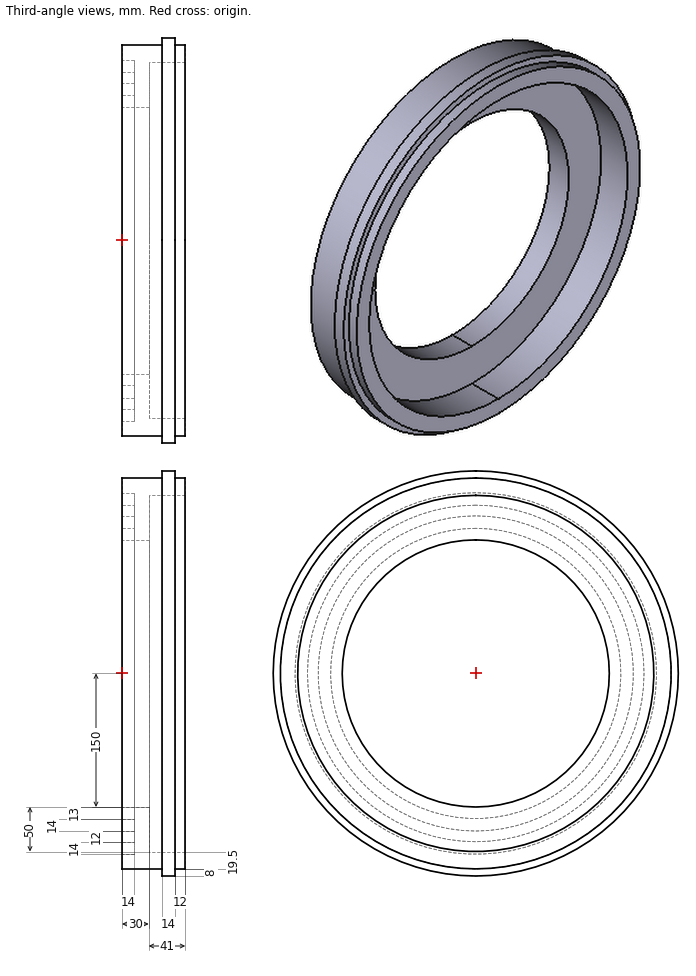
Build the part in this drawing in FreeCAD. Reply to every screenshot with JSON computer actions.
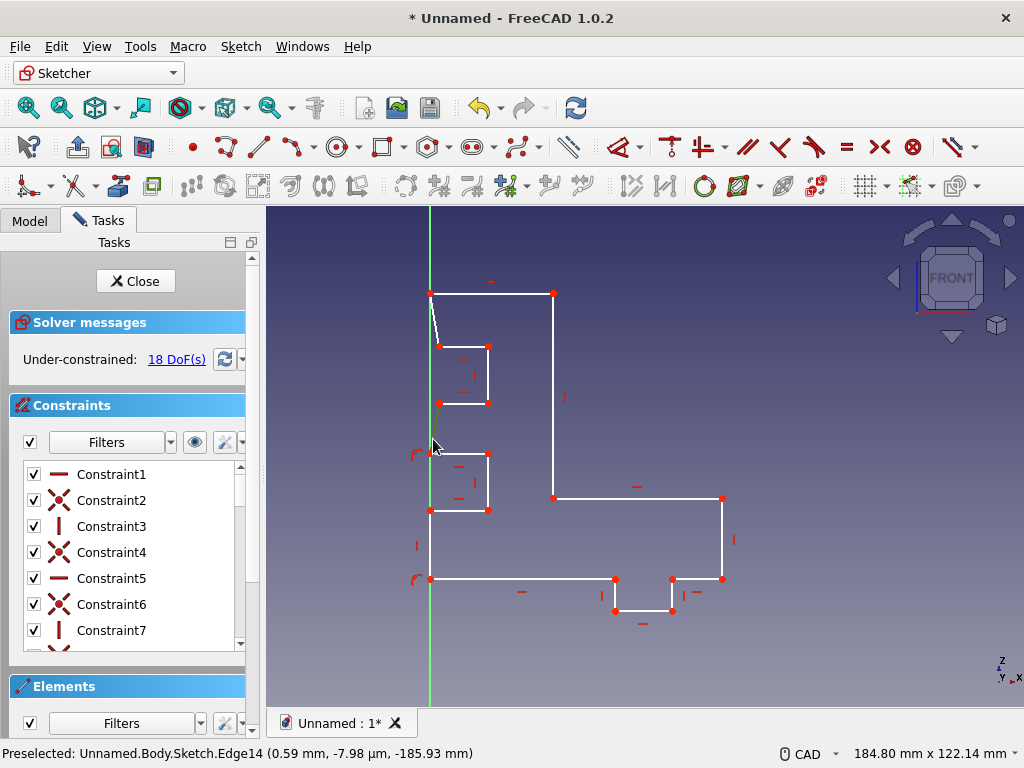
{"action": "left_click", "coordinate": [724, 148]}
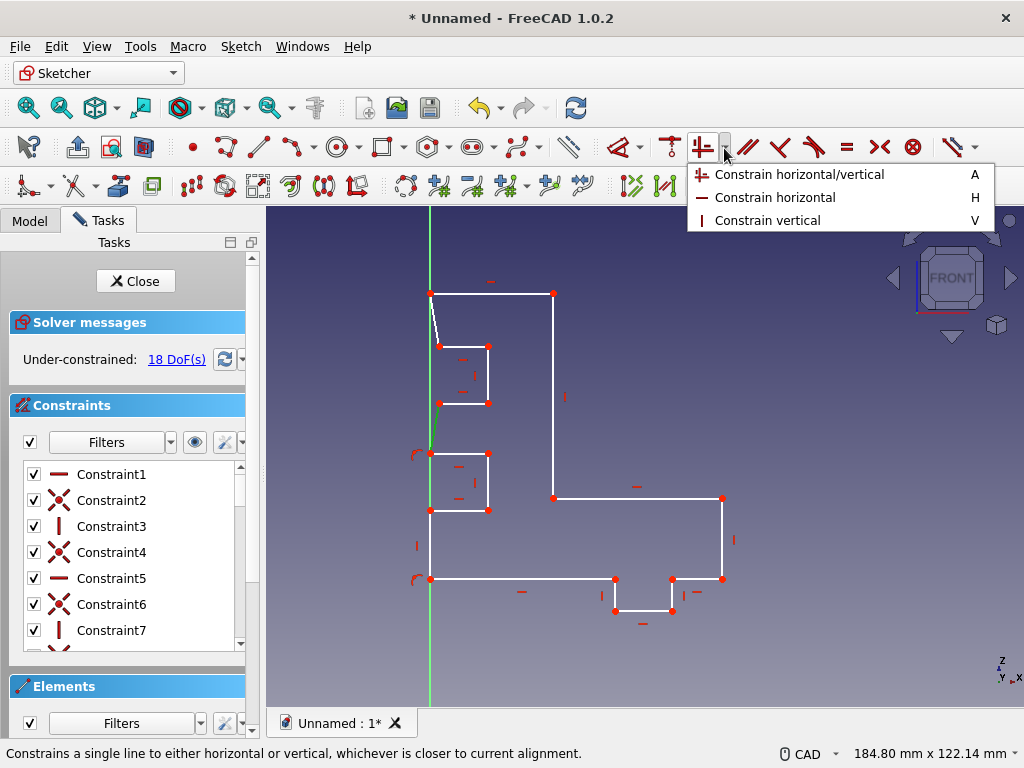
{"action": "left_click", "coordinate": [841, 220]}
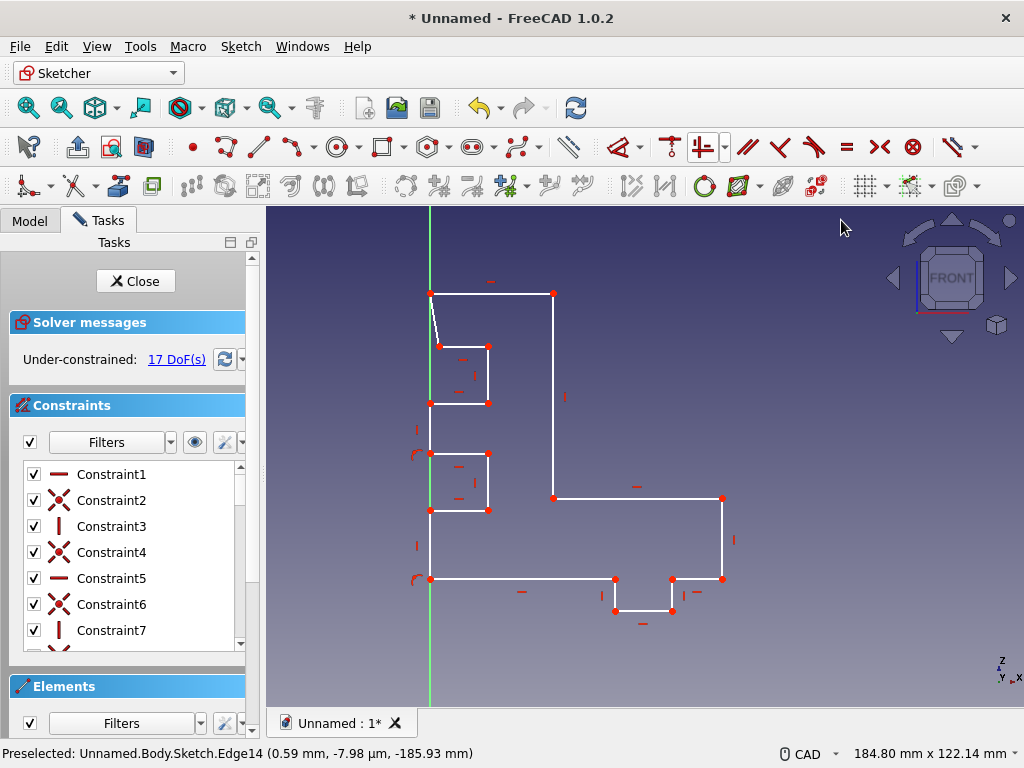
{"action": "left_click", "coordinate": [433, 310]}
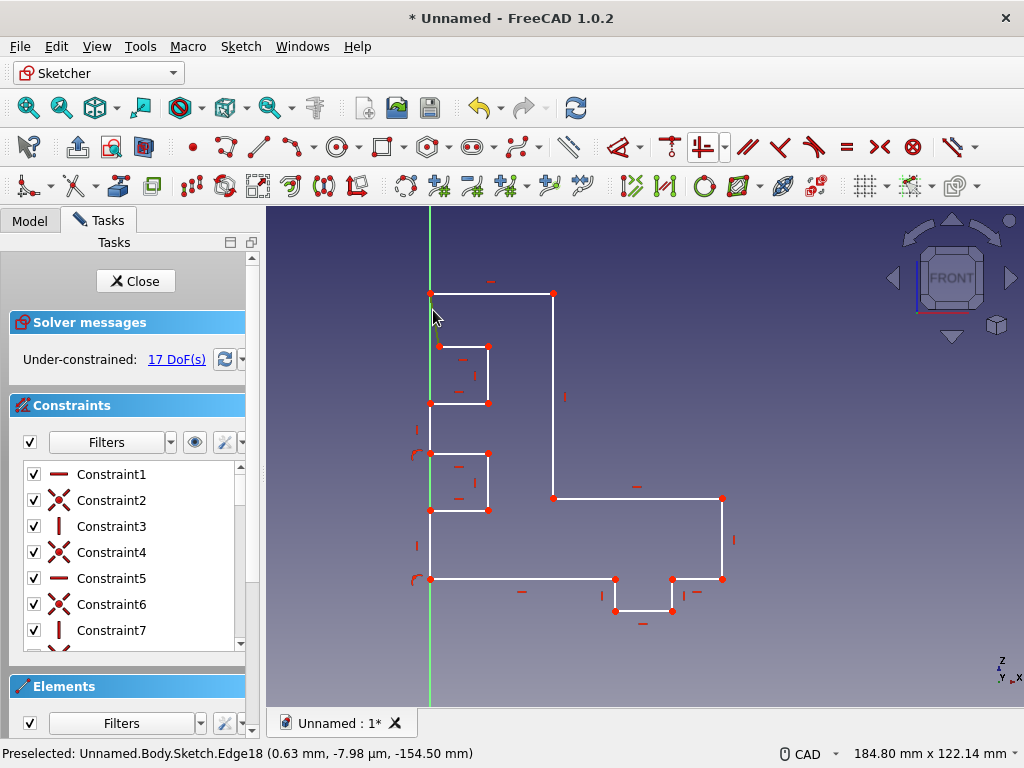
{"action": "key", "text": "v"}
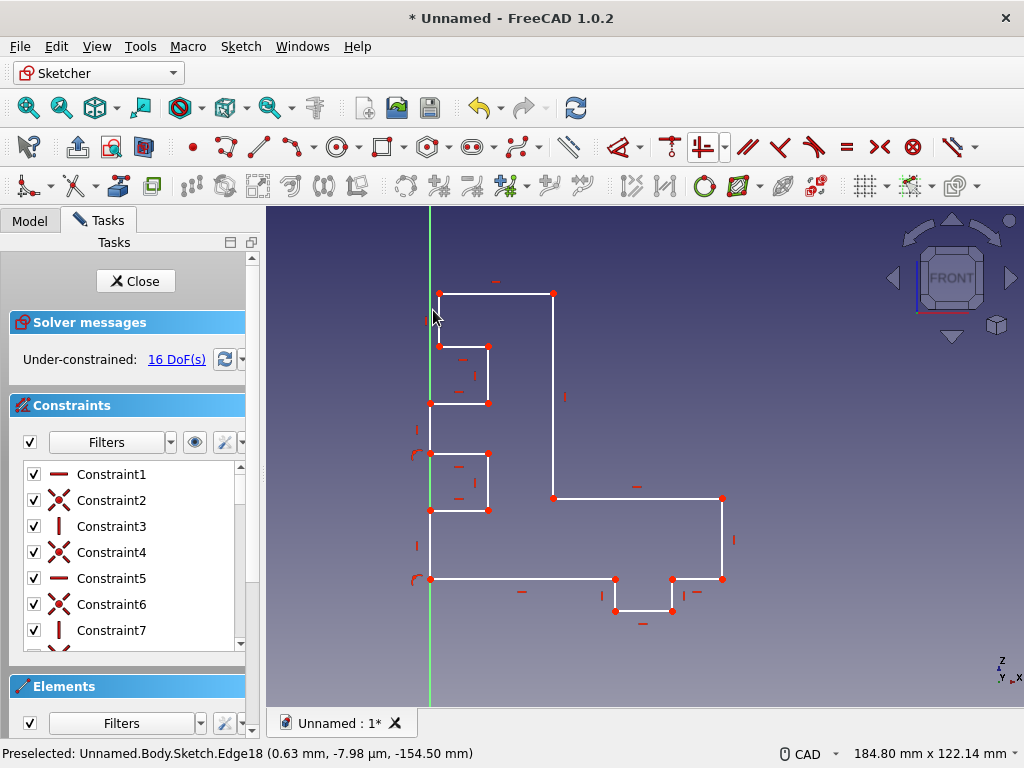
{"action": "left_click", "coordinate": [439, 294]}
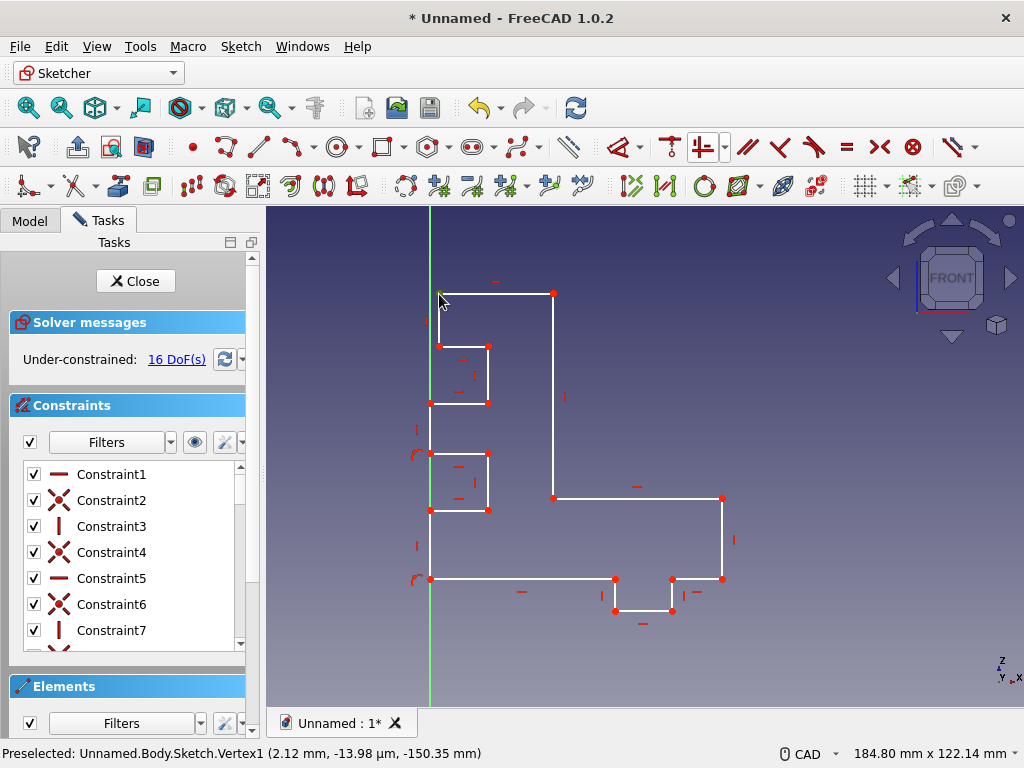
{"action": "left_click", "coordinate": [430, 647]}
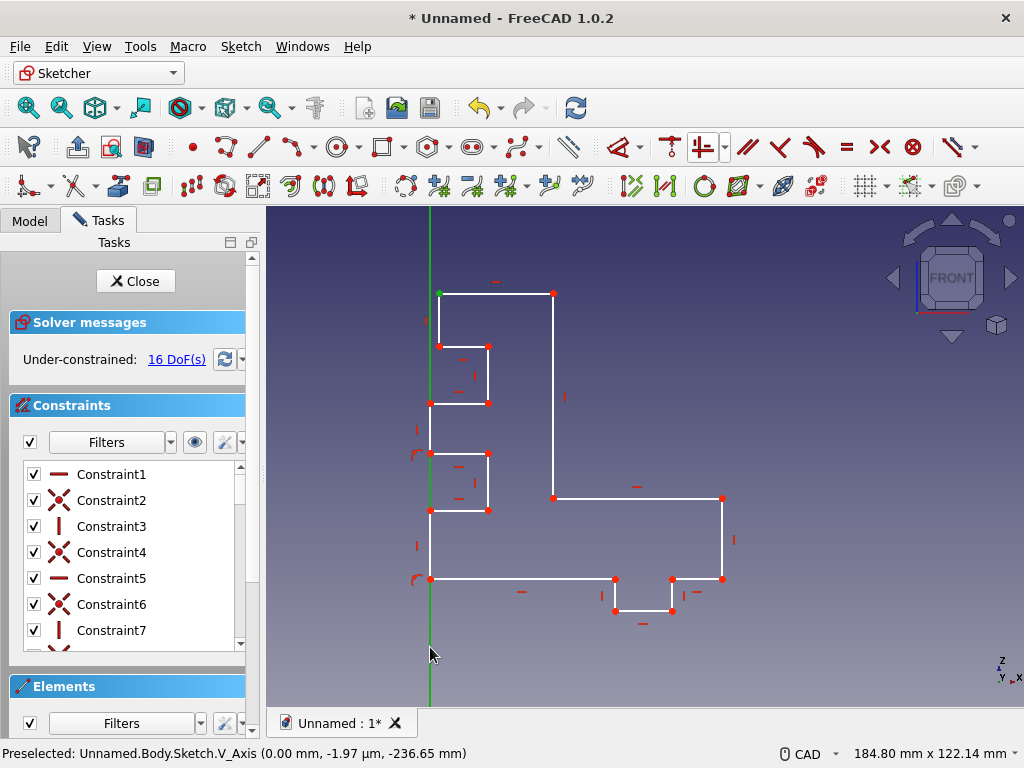
{"action": "left_click", "coordinate": [670, 148]}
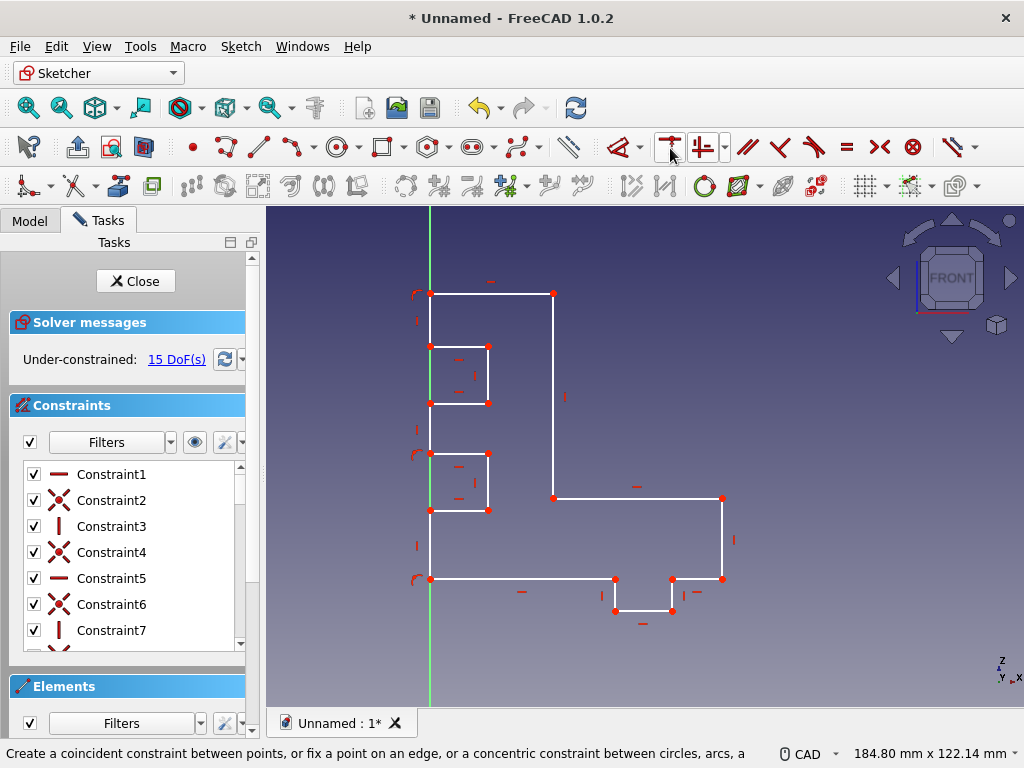
{"action": "left_click", "coordinate": [618, 148]}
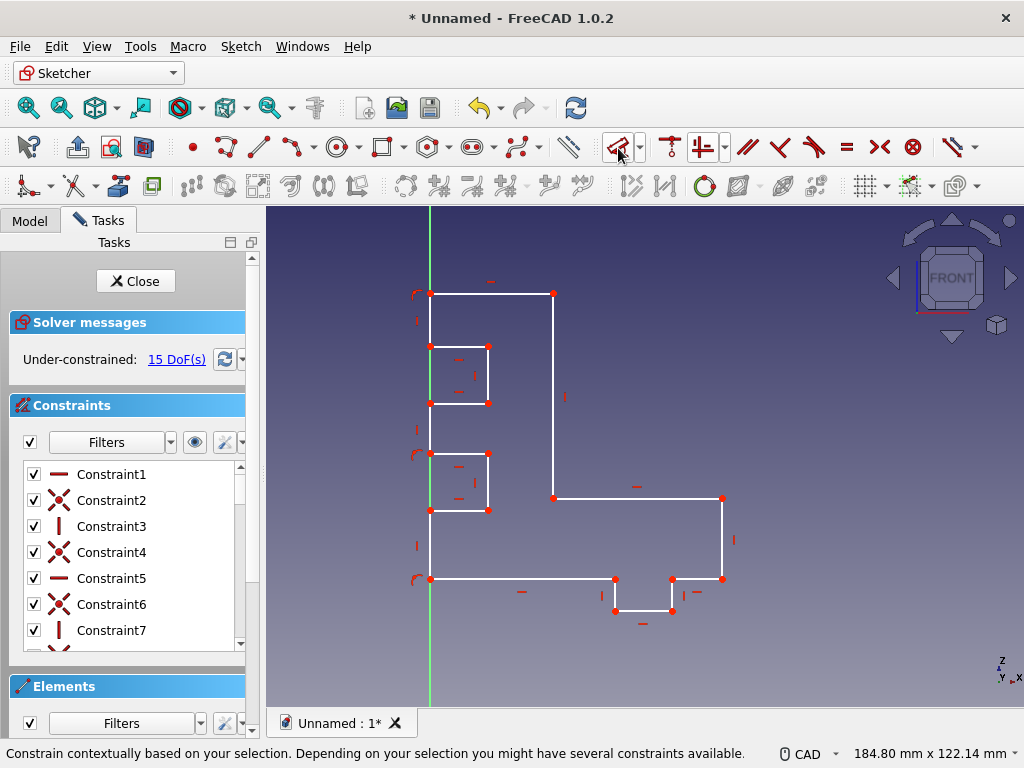
{"action": "scroll", "coordinate": [672, 589], "scroll_direction": "up", "scroll_amount": 2}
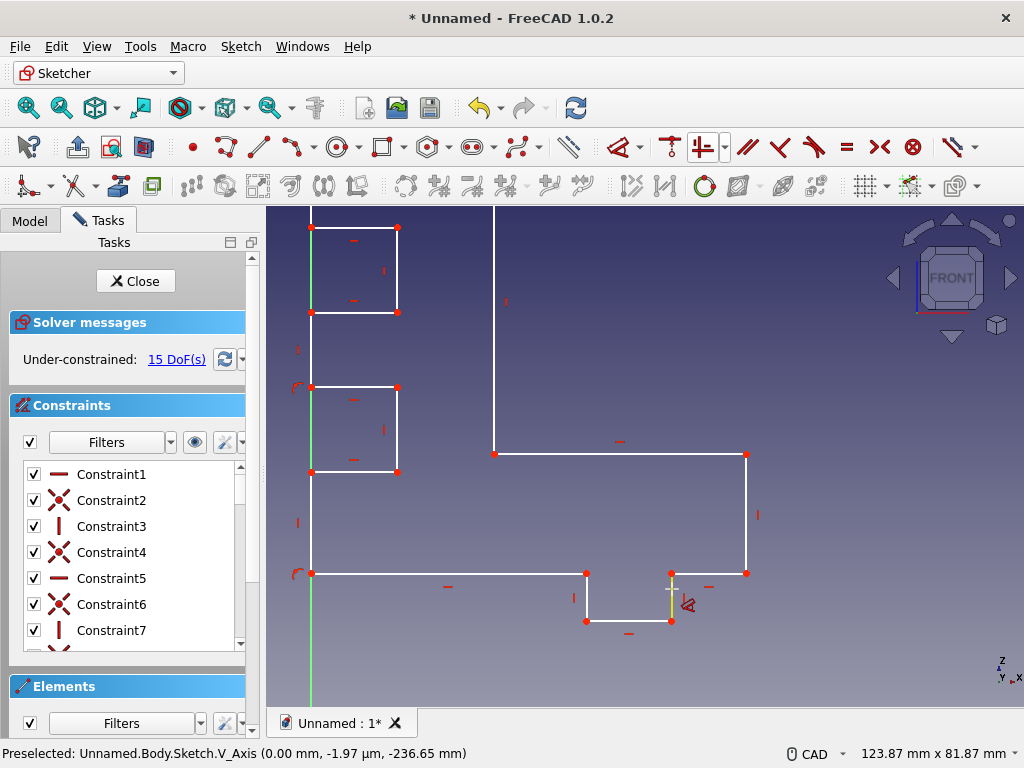
{"action": "left_click", "coordinate": [672, 588]}
{"action": "left_click", "coordinate": [706, 598]}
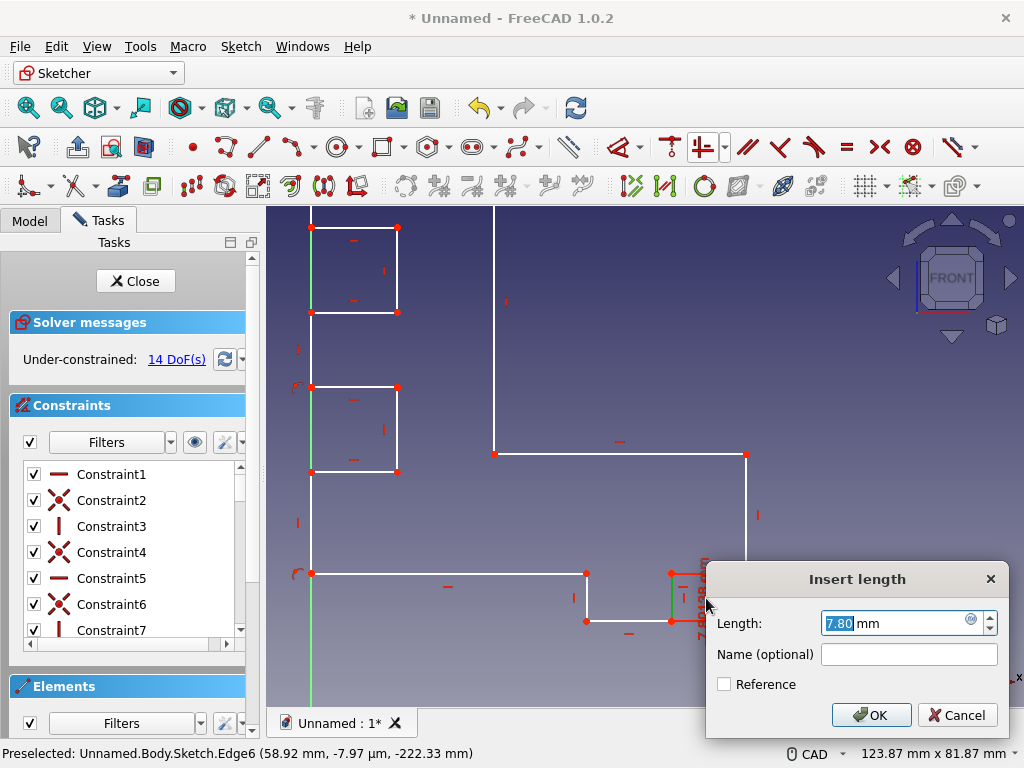
{"action": "type", "text": "8"}
{"action": "key", "text": "Return"}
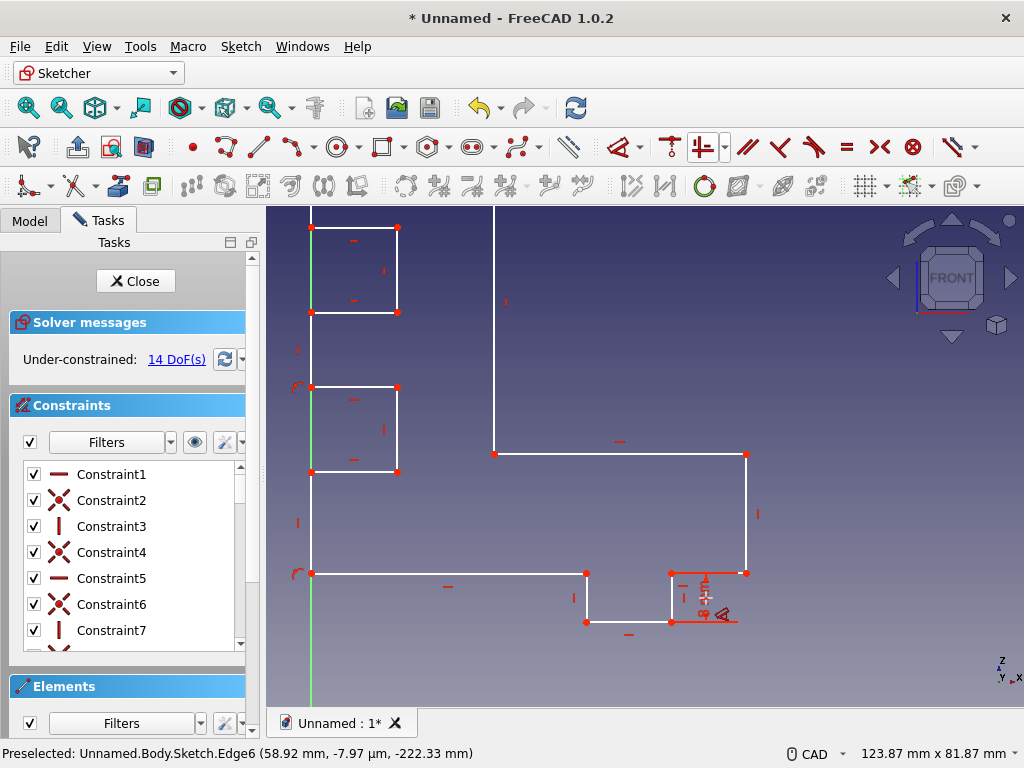
{"action": "left_click", "coordinate": [587, 608]}
{"action": "left_click", "coordinate": [621, 598]}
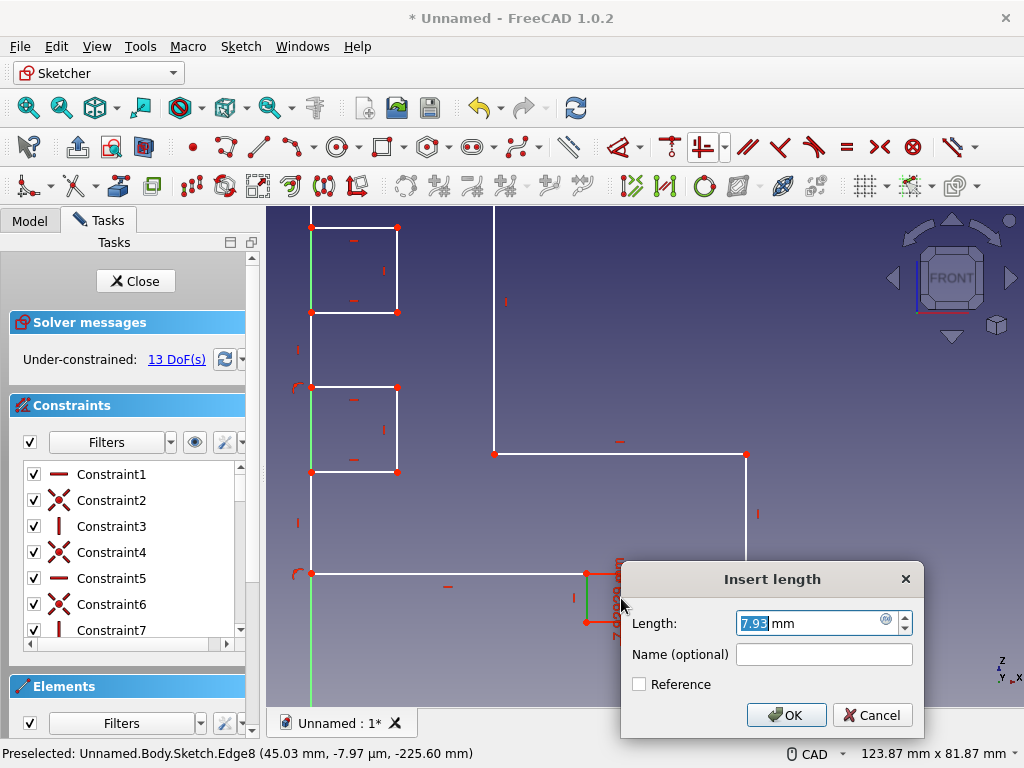
{"action": "type", "text": "8"}
{"action": "key", "text": "Return"}